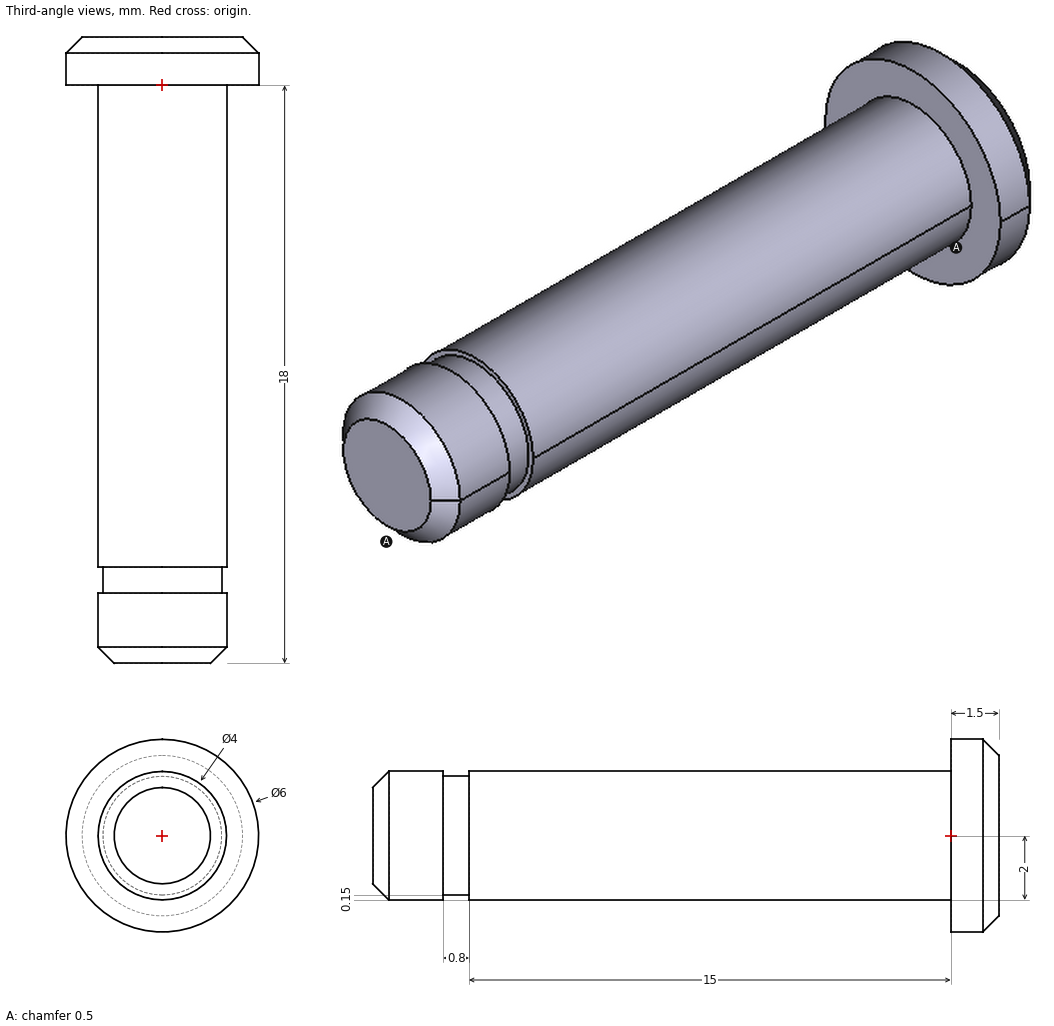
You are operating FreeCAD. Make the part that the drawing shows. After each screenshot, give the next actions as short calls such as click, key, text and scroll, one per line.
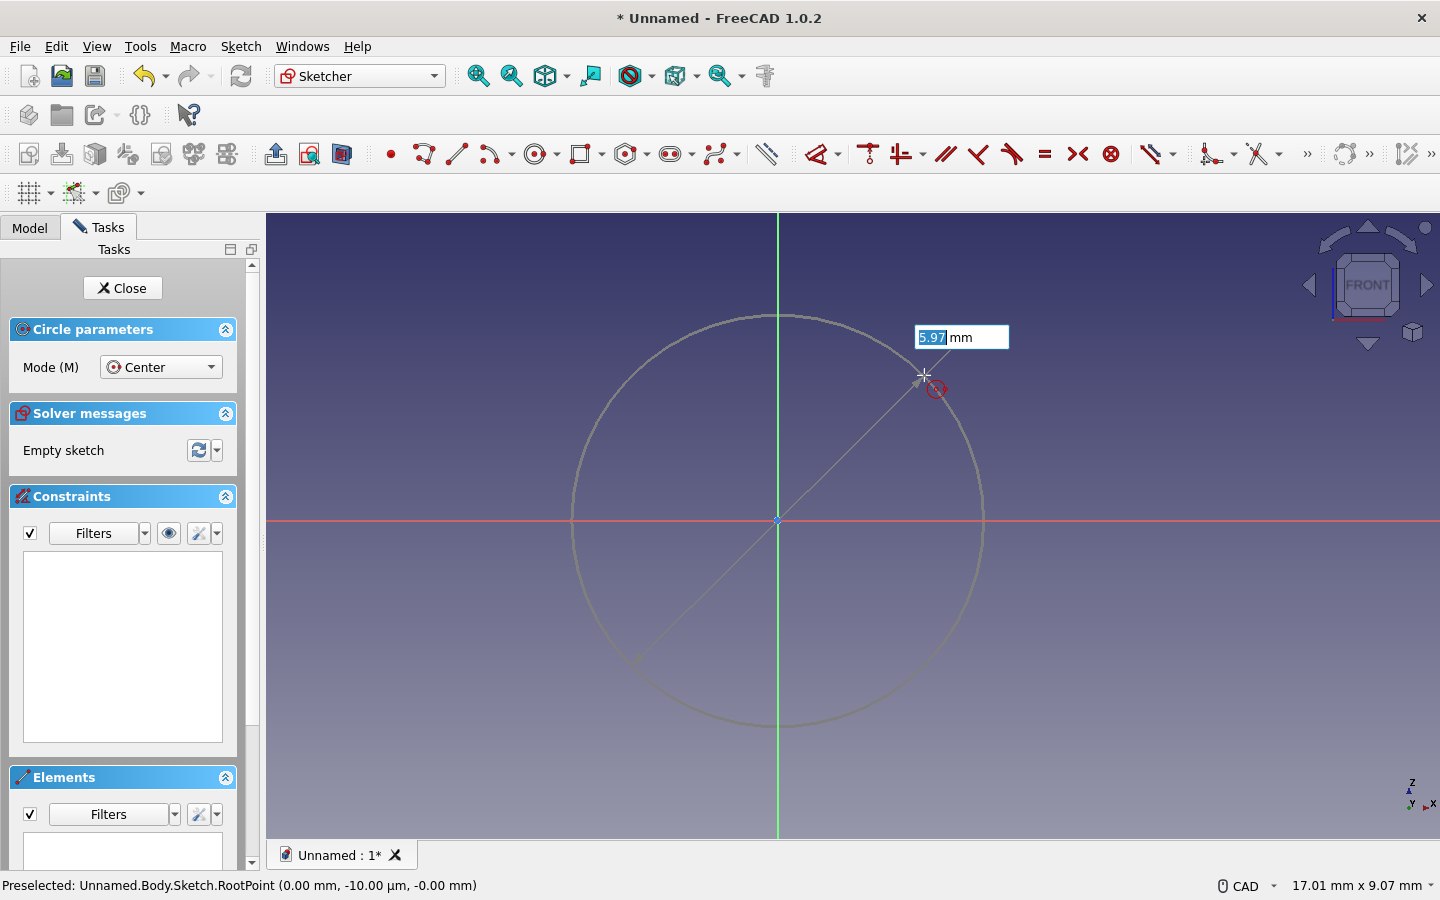
text(6)
key(Return)
key(Escape)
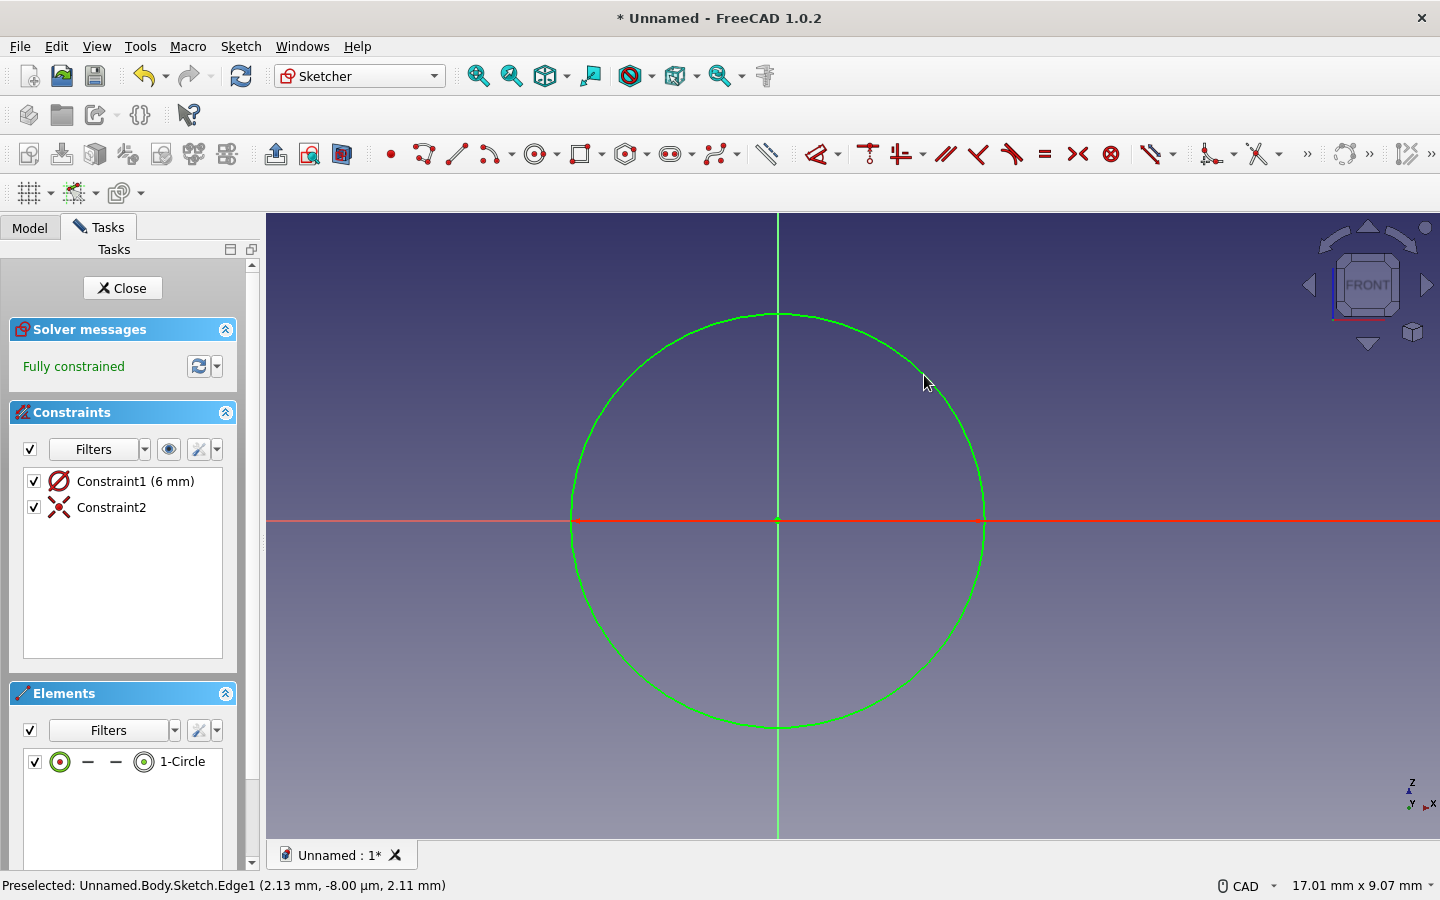
click(123, 288)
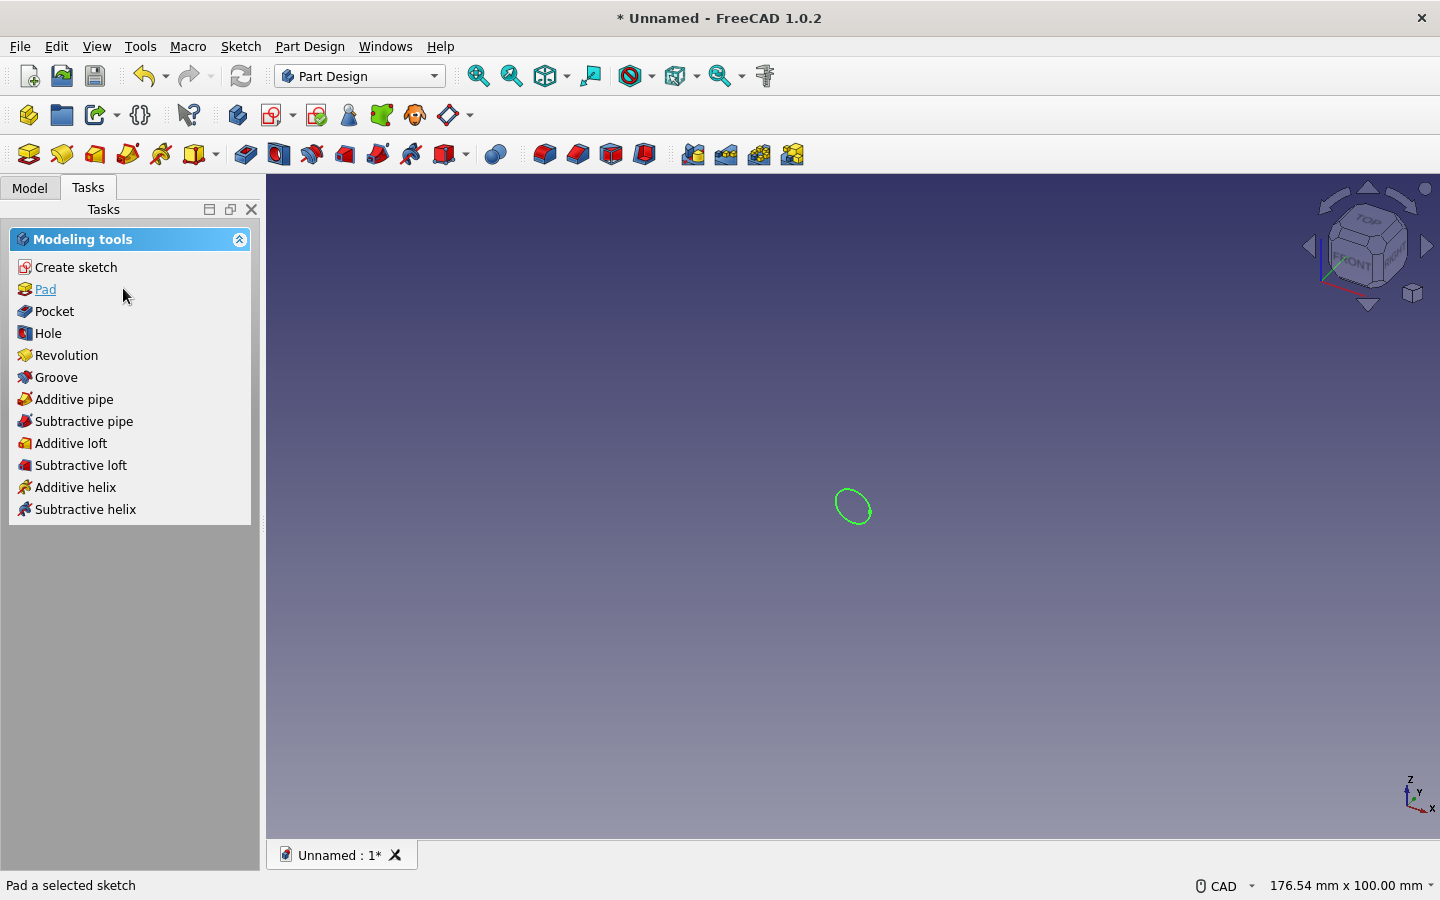
click(29, 154)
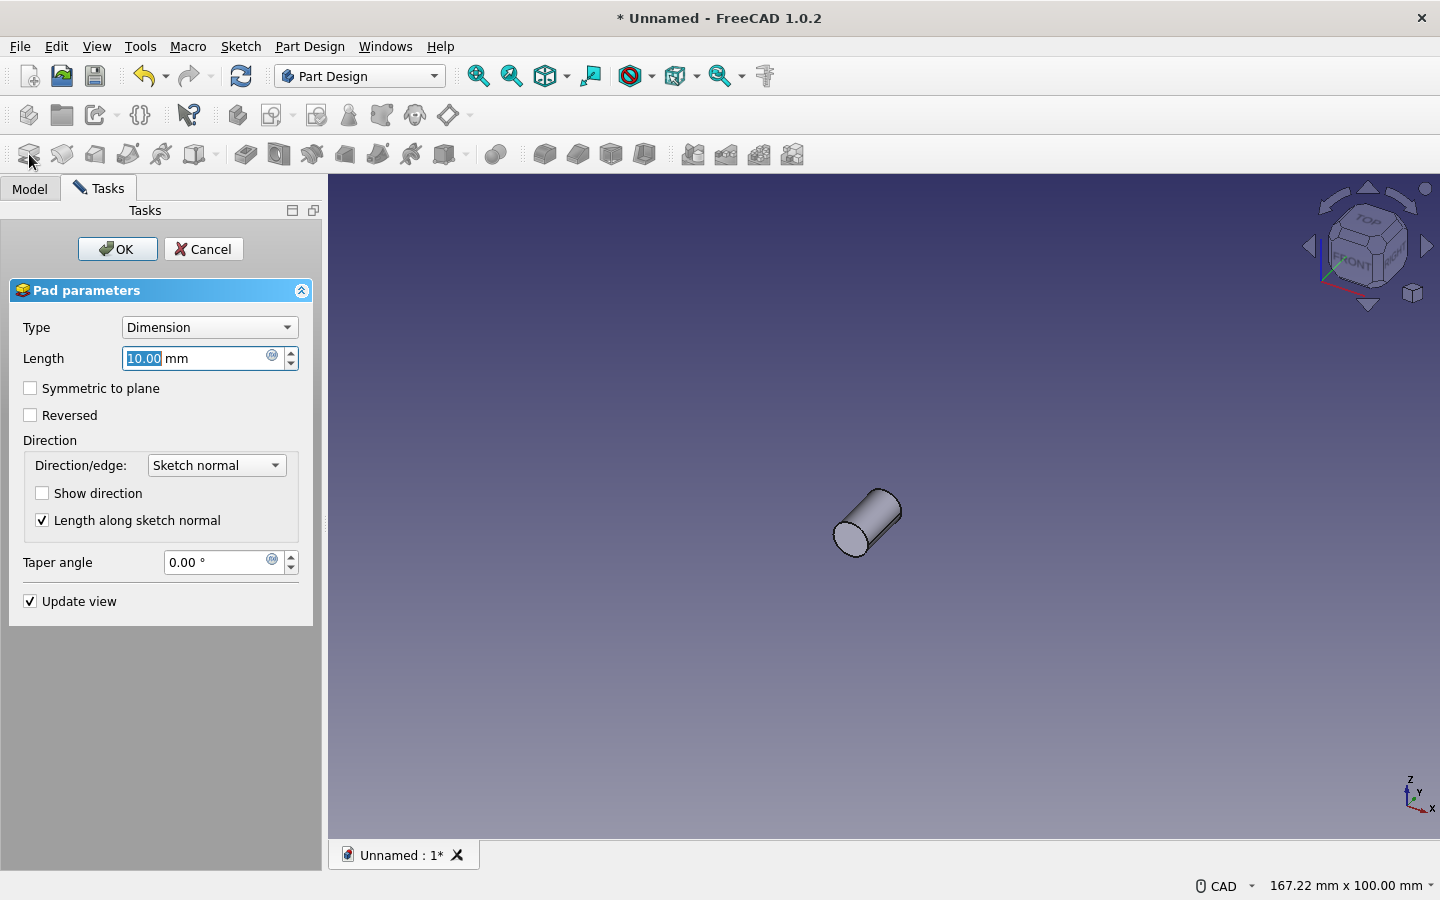
text(1.5)
key(Tab)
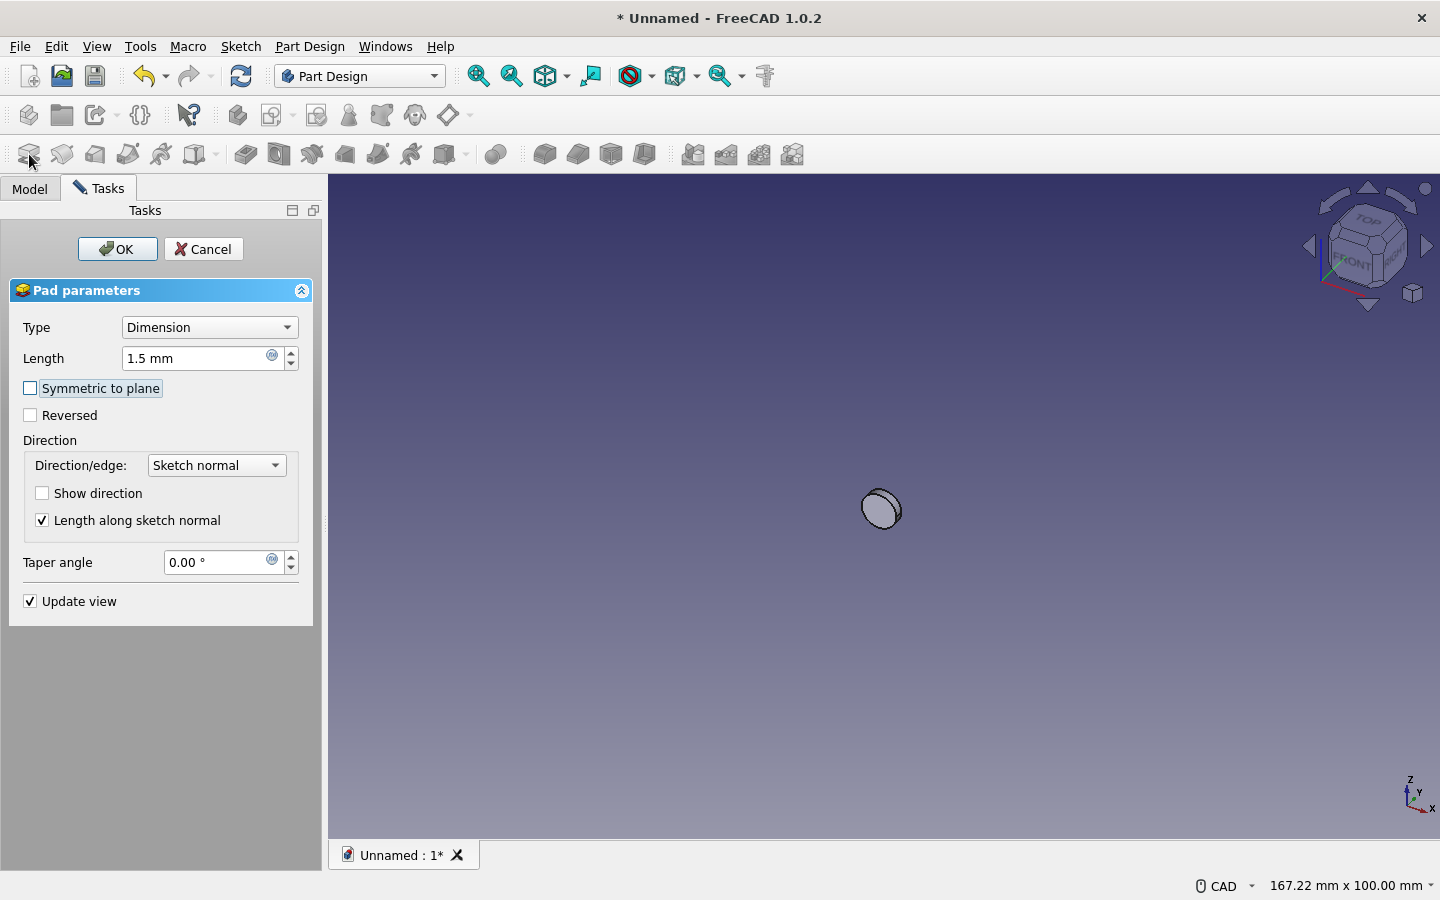
click(31, 415)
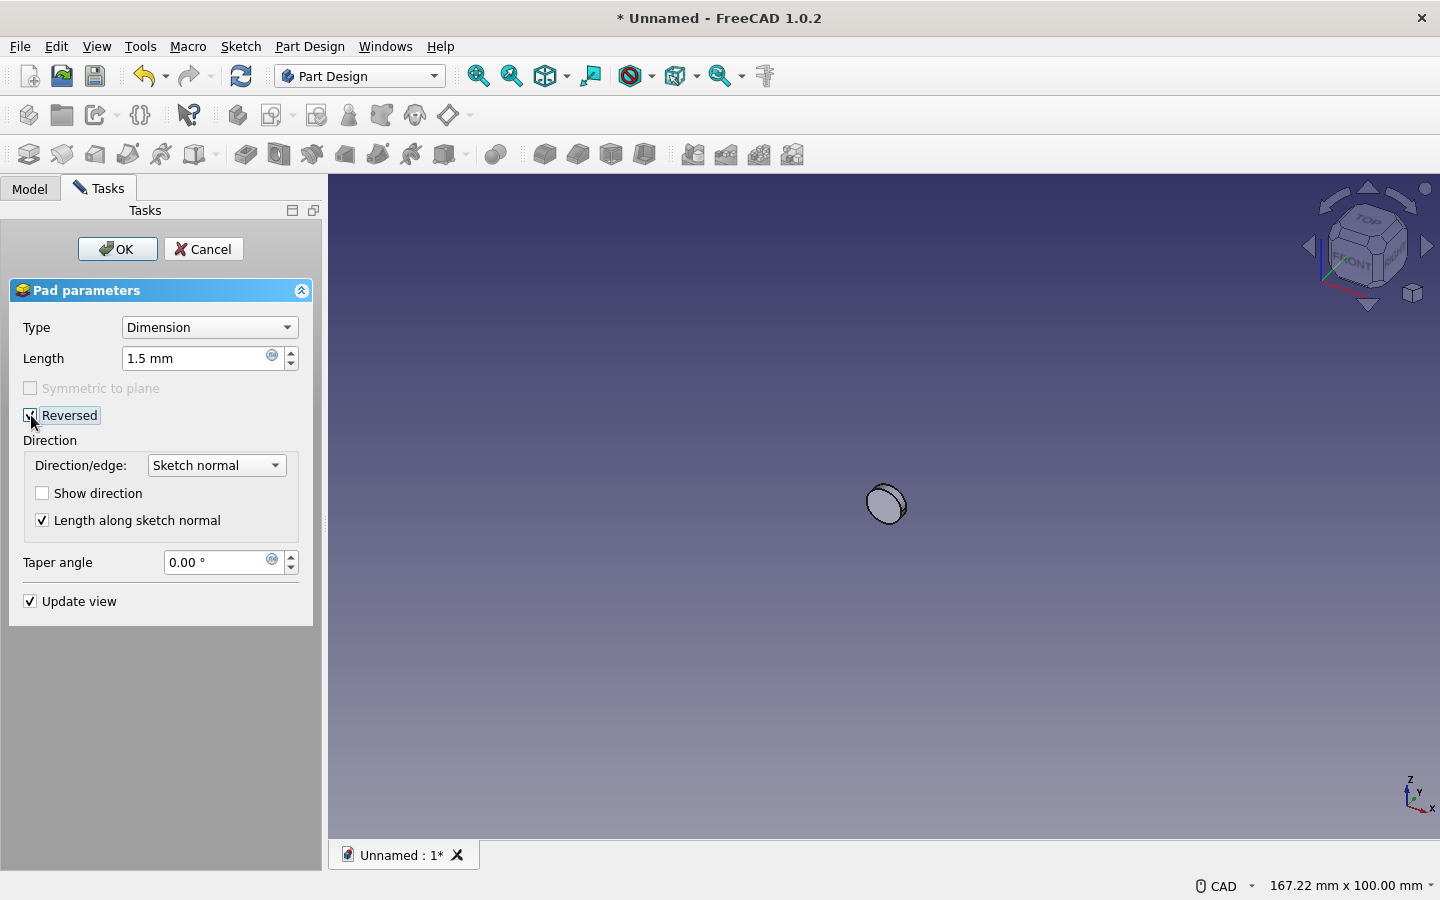
click(118, 249)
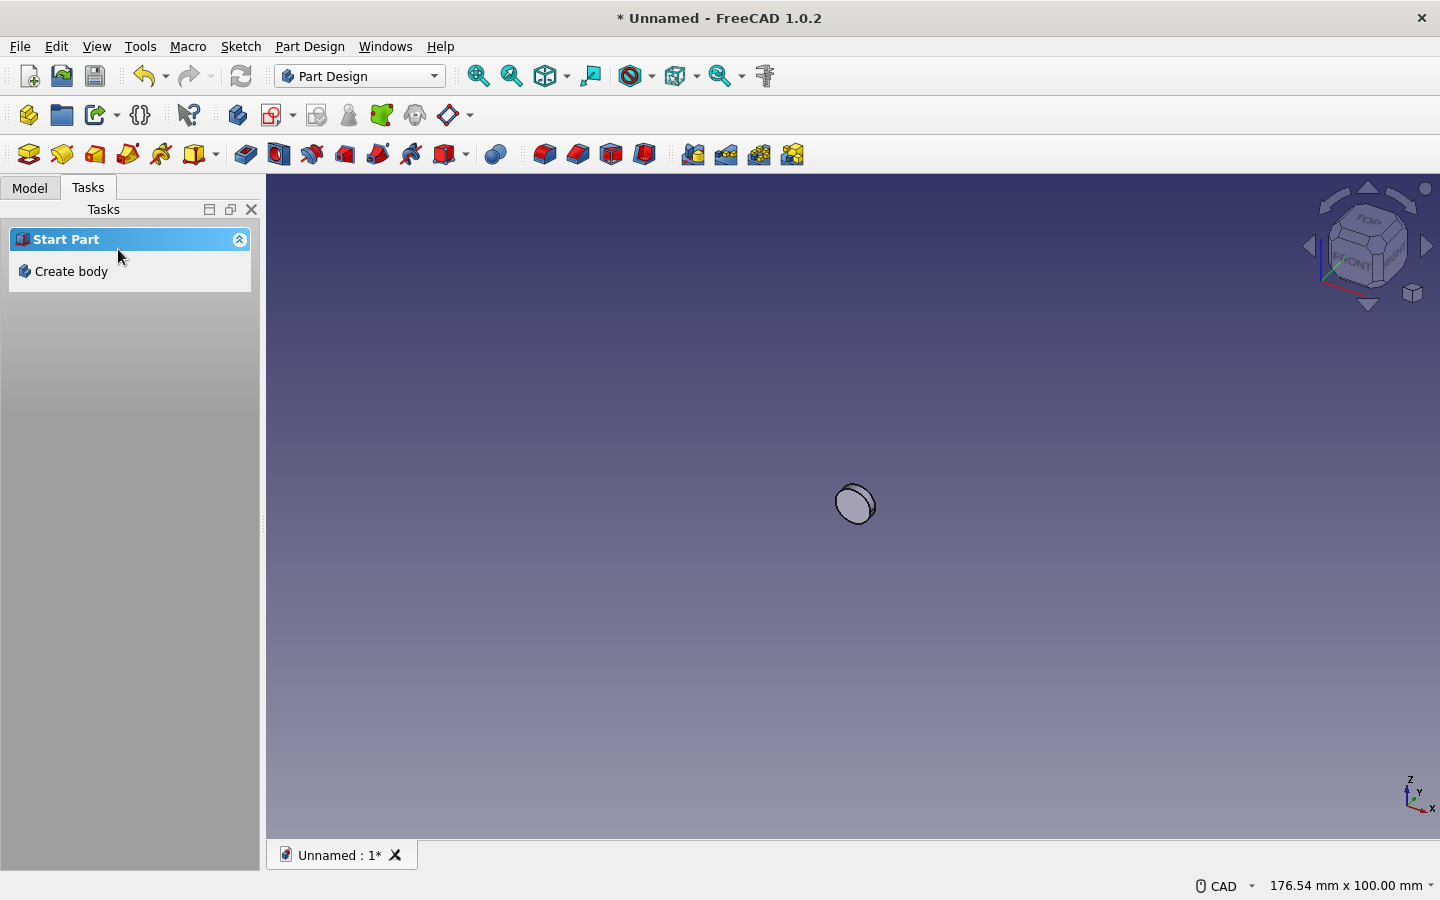
key(v)
key(f)